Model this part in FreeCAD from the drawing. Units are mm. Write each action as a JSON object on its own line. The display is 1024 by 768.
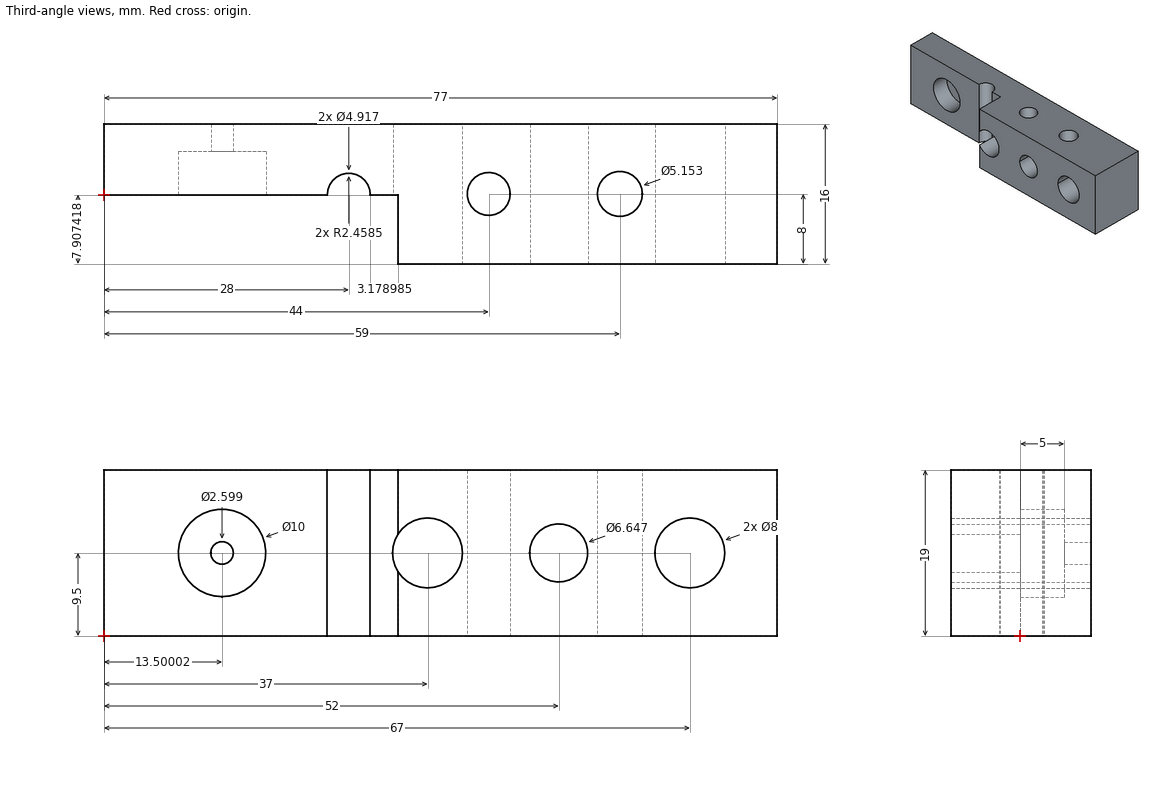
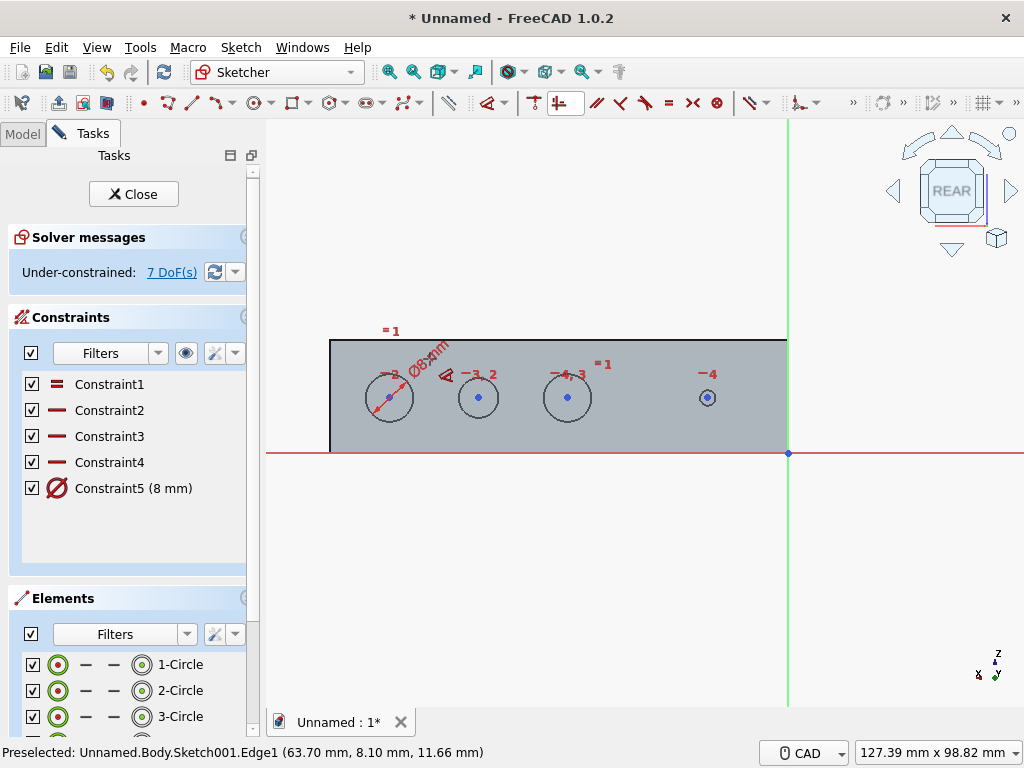
{"action": "left_click", "coordinate": [493, 384]}
{"action": "left_click", "coordinate": [516, 362]}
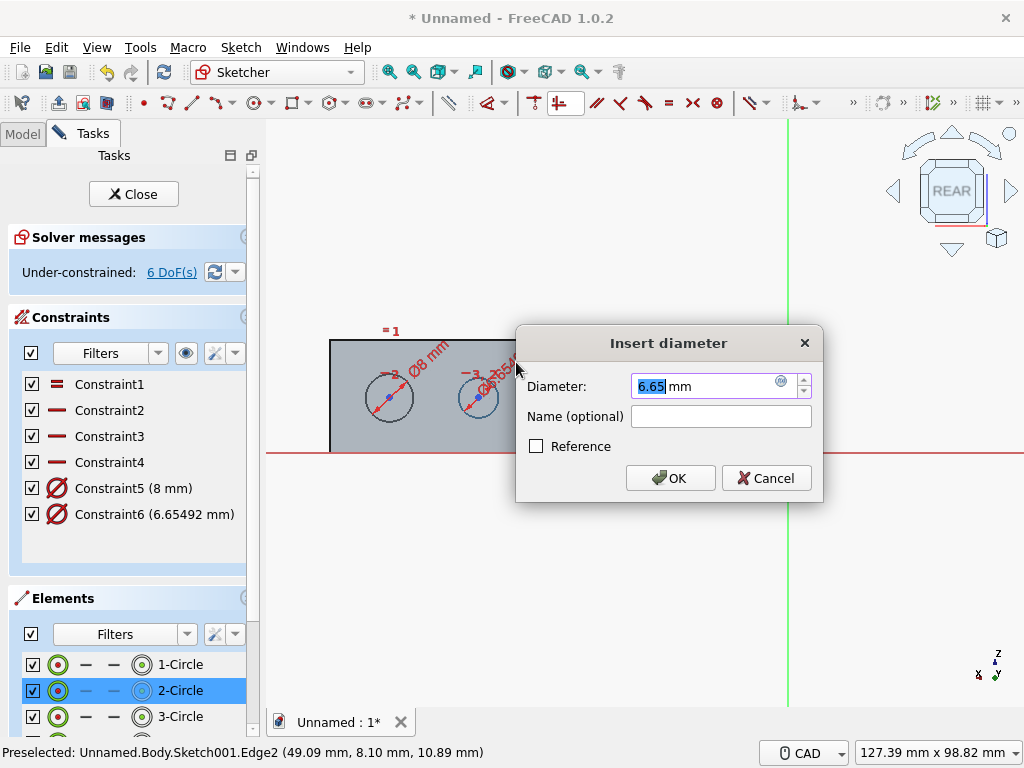
{"action": "type", "text": "6.647"}
{"action": "key", "text": "Return"}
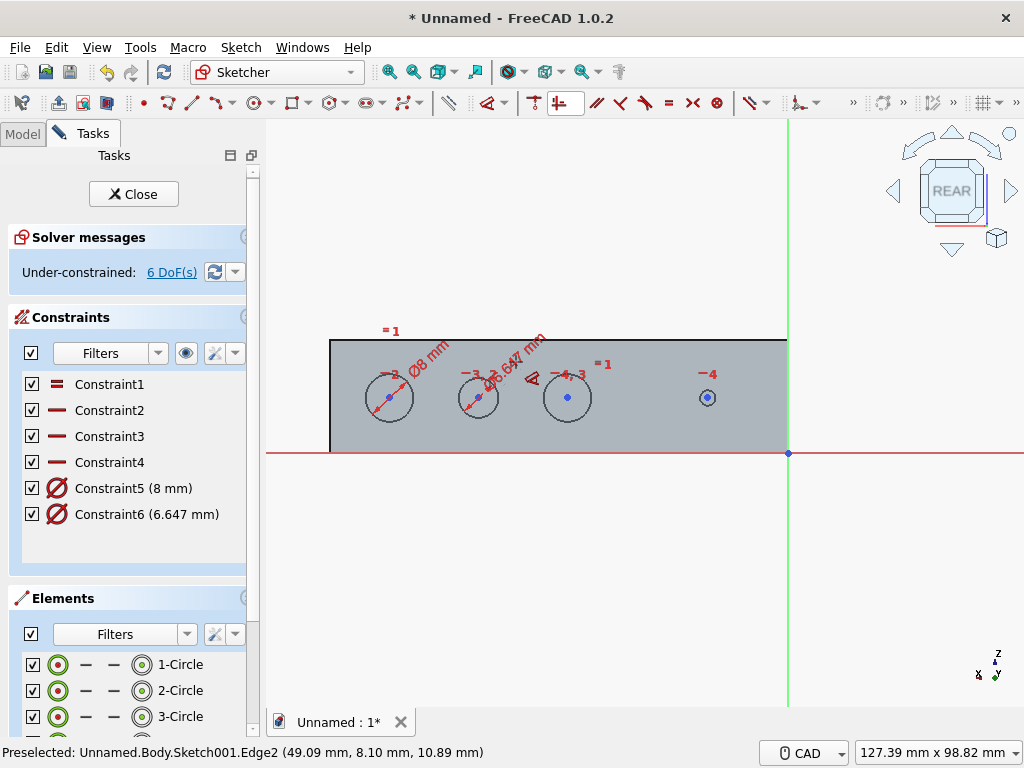
{"action": "scroll", "coordinate": [702, 393], "scroll_direction": "up", "scroll_amount": 5}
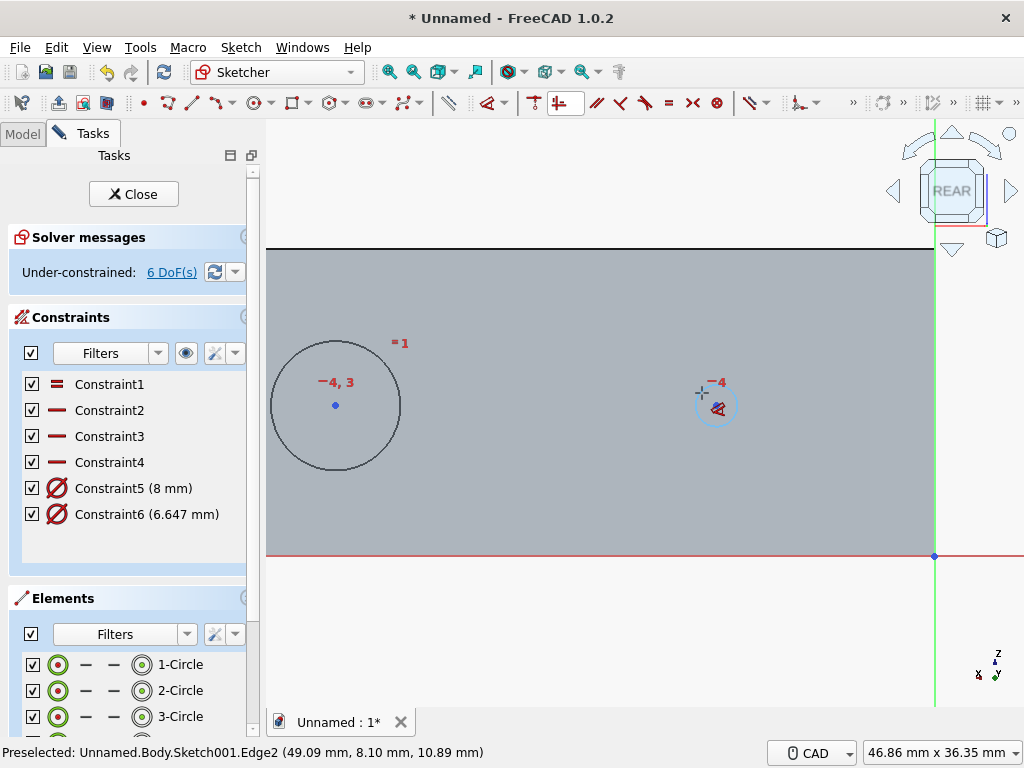
{"action": "left_click", "coordinate": [702, 391]}
{"action": "left_click", "coordinate": [680, 368]}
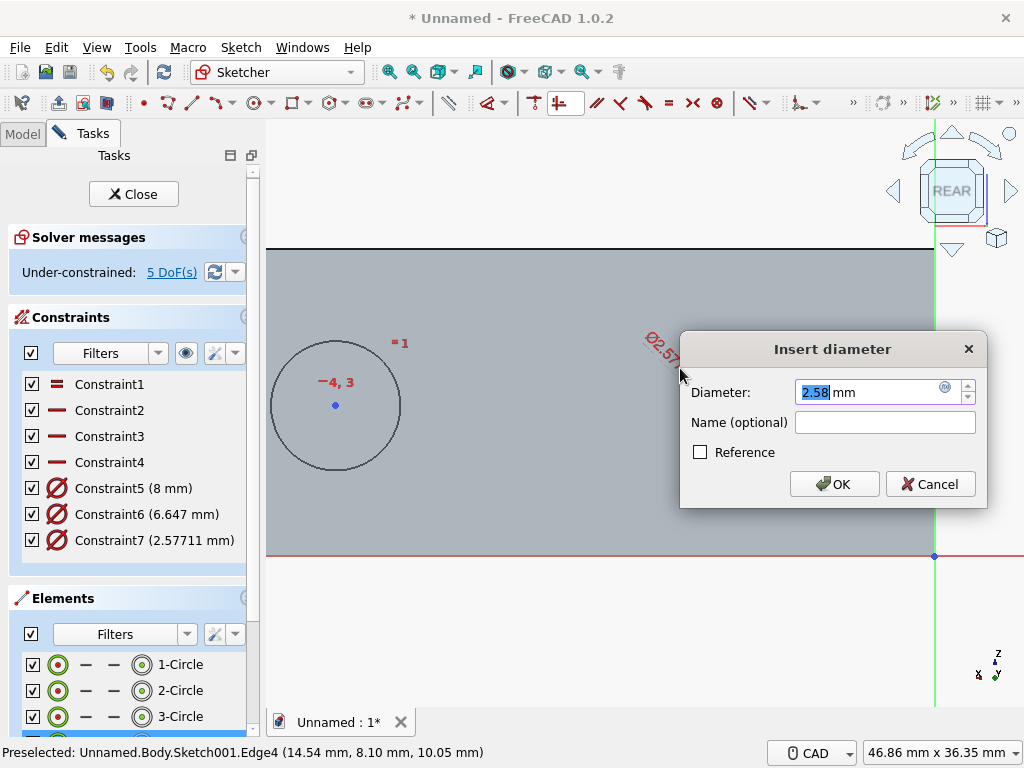
{"action": "type", "text": "2.599"}
{"action": "key", "text": "Return"}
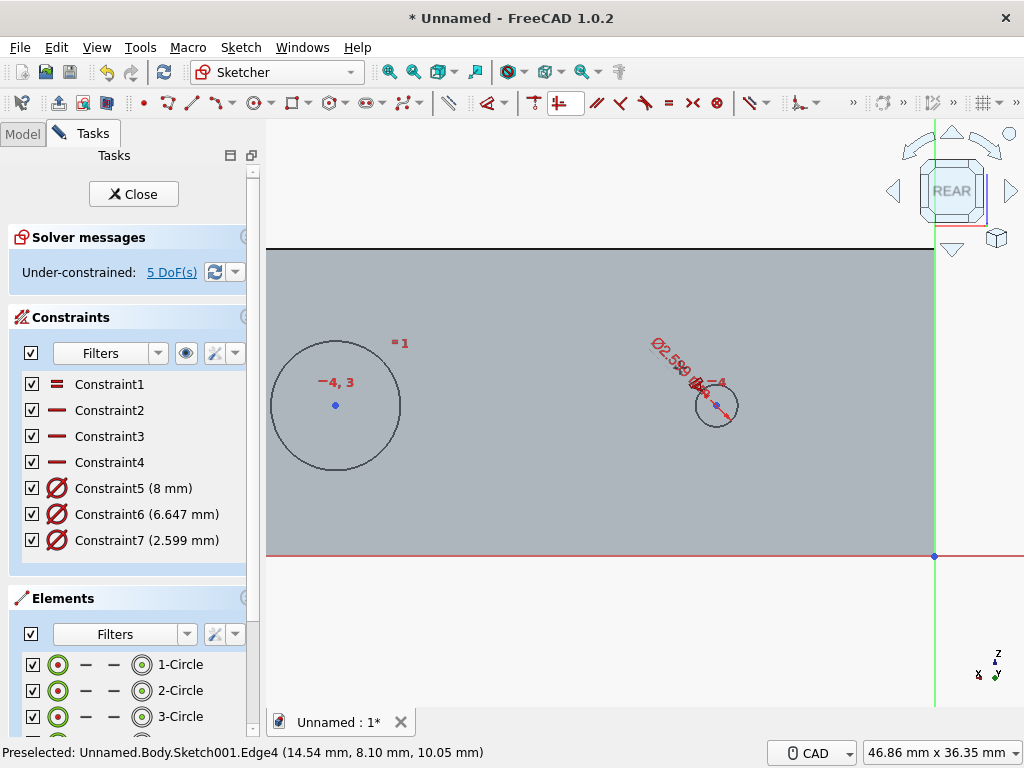
{"action": "scroll", "coordinate": [702, 393], "scroll_direction": "down", "scroll_amount": 5}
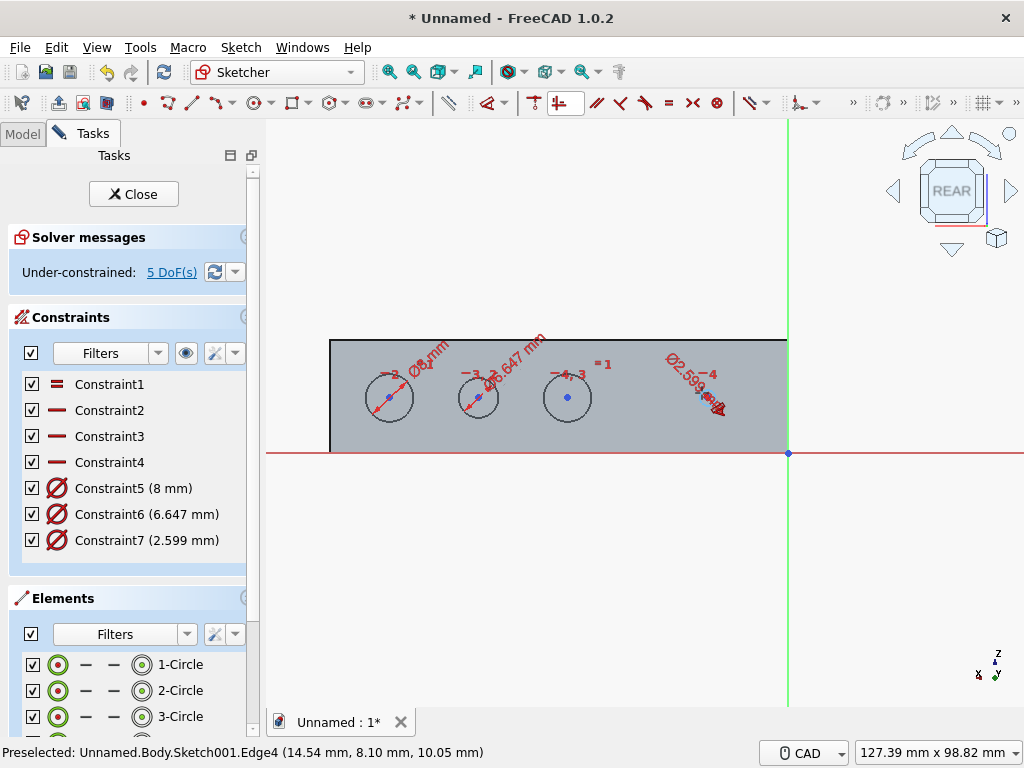
{"action": "left_click", "coordinate": [390, 398]}
{"action": "left_click", "coordinate": [589, 487]}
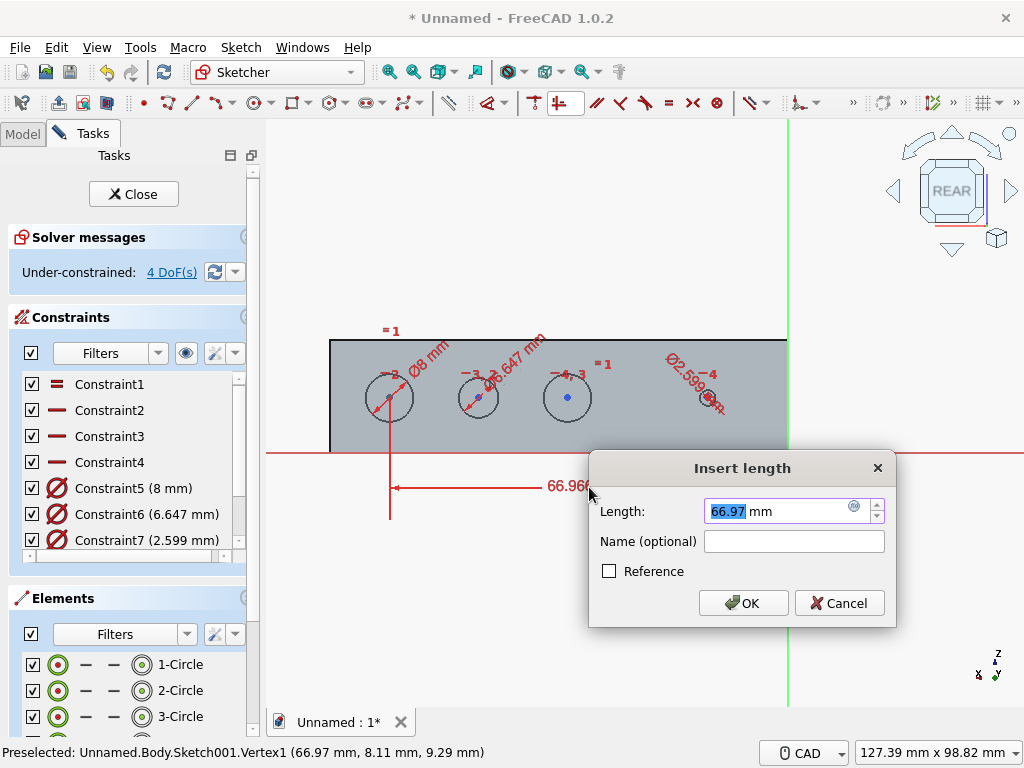
{"action": "type", "text": "67"}
{"action": "key", "text": "Return"}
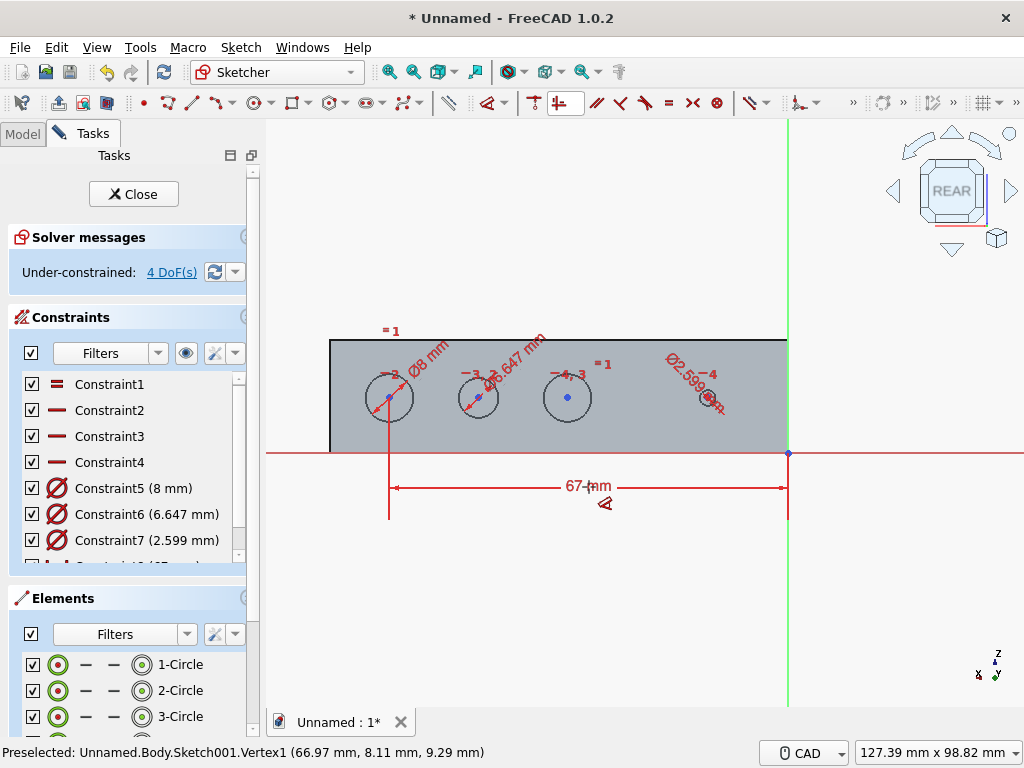
{"action": "left_click", "coordinate": [479, 398]}
{"action": "left_click", "coordinate": [705, 487]}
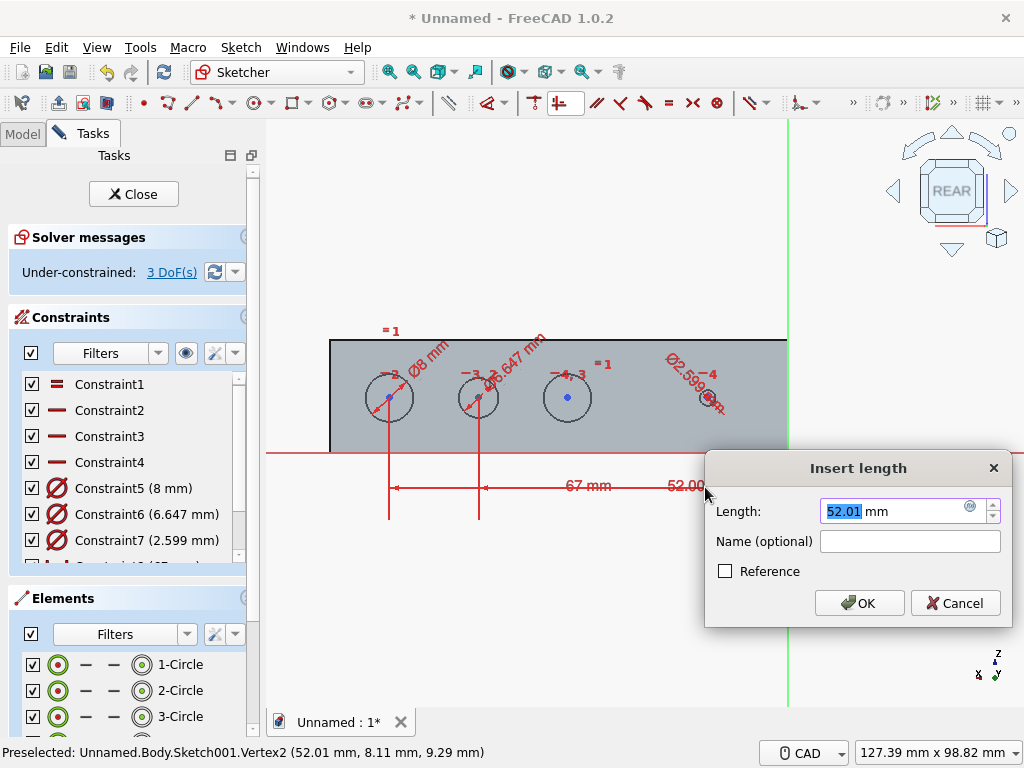
{"action": "type", "text": "52"}
{"action": "key", "text": "Return"}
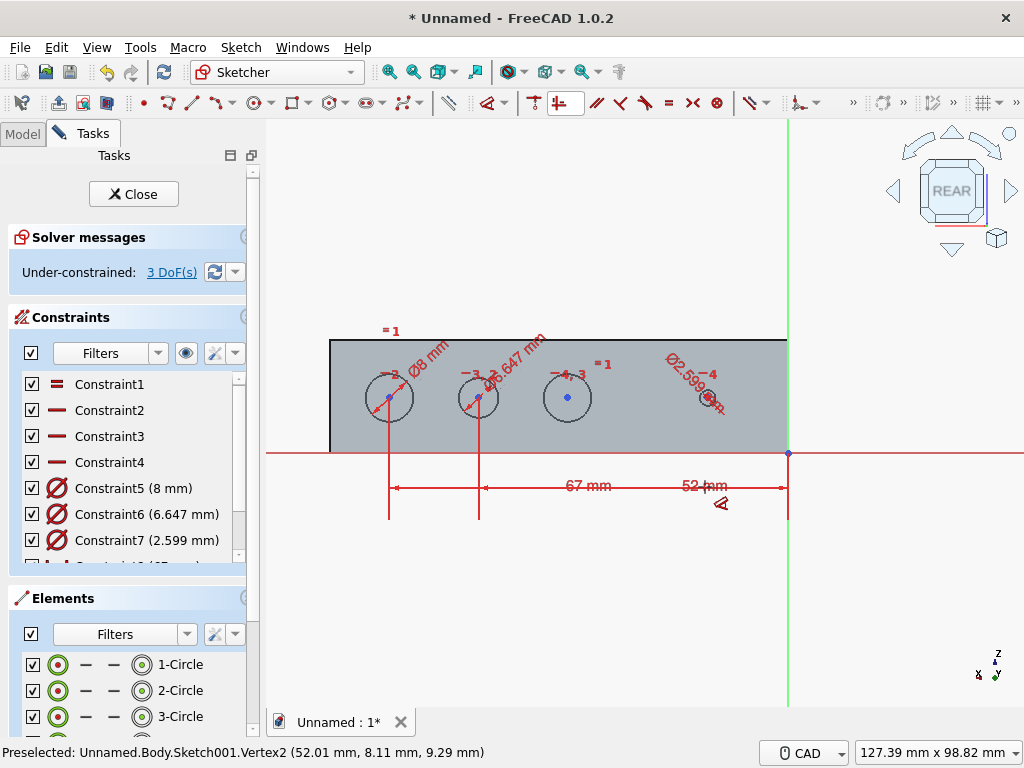
{"action": "left_click", "coordinate": [568, 398]}
{"action": "left_click", "coordinate": [678, 364]}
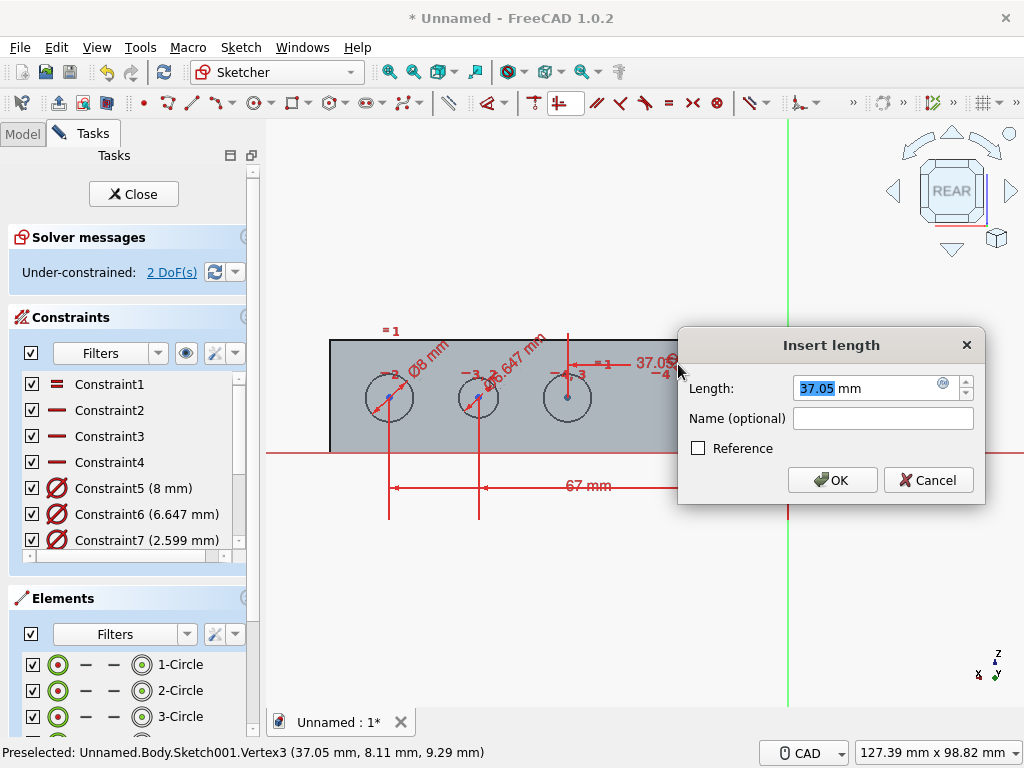
{"action": "type", "text": "37"}
{"action": "key", "text": "Return"}